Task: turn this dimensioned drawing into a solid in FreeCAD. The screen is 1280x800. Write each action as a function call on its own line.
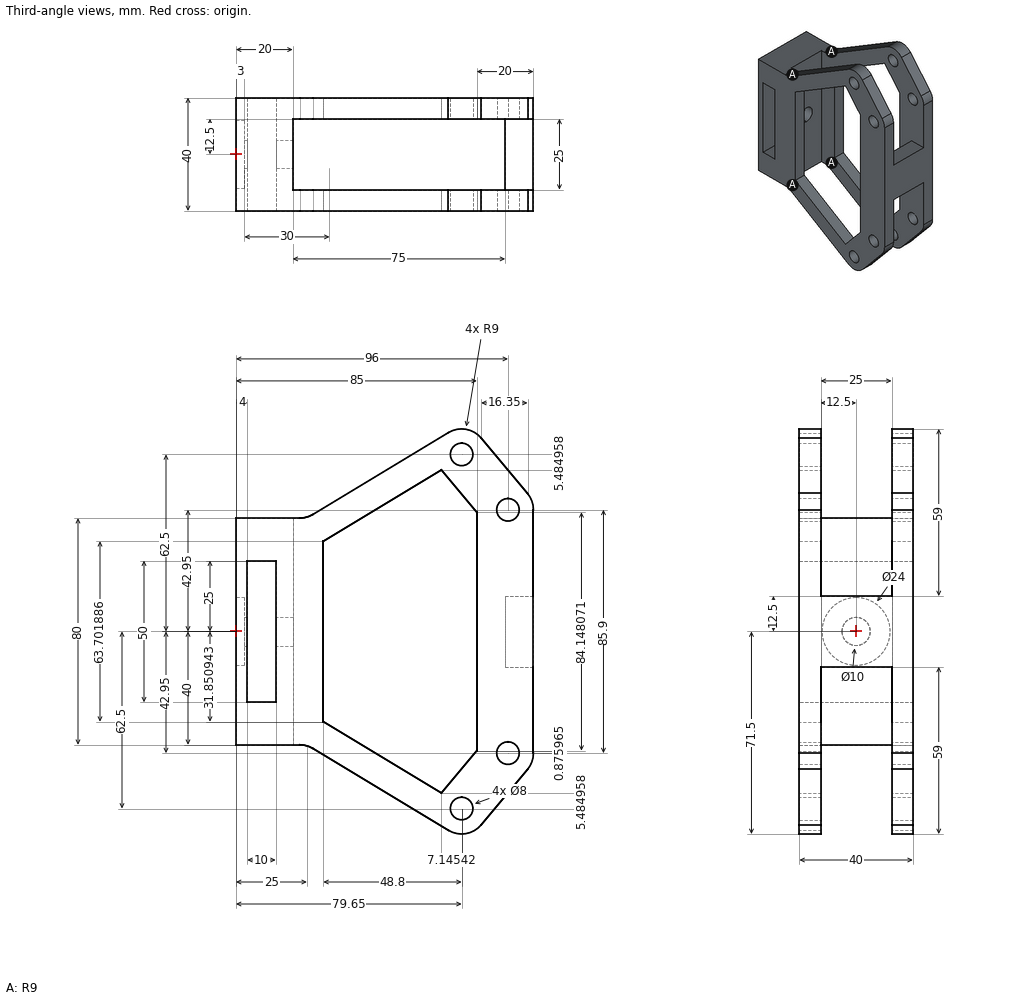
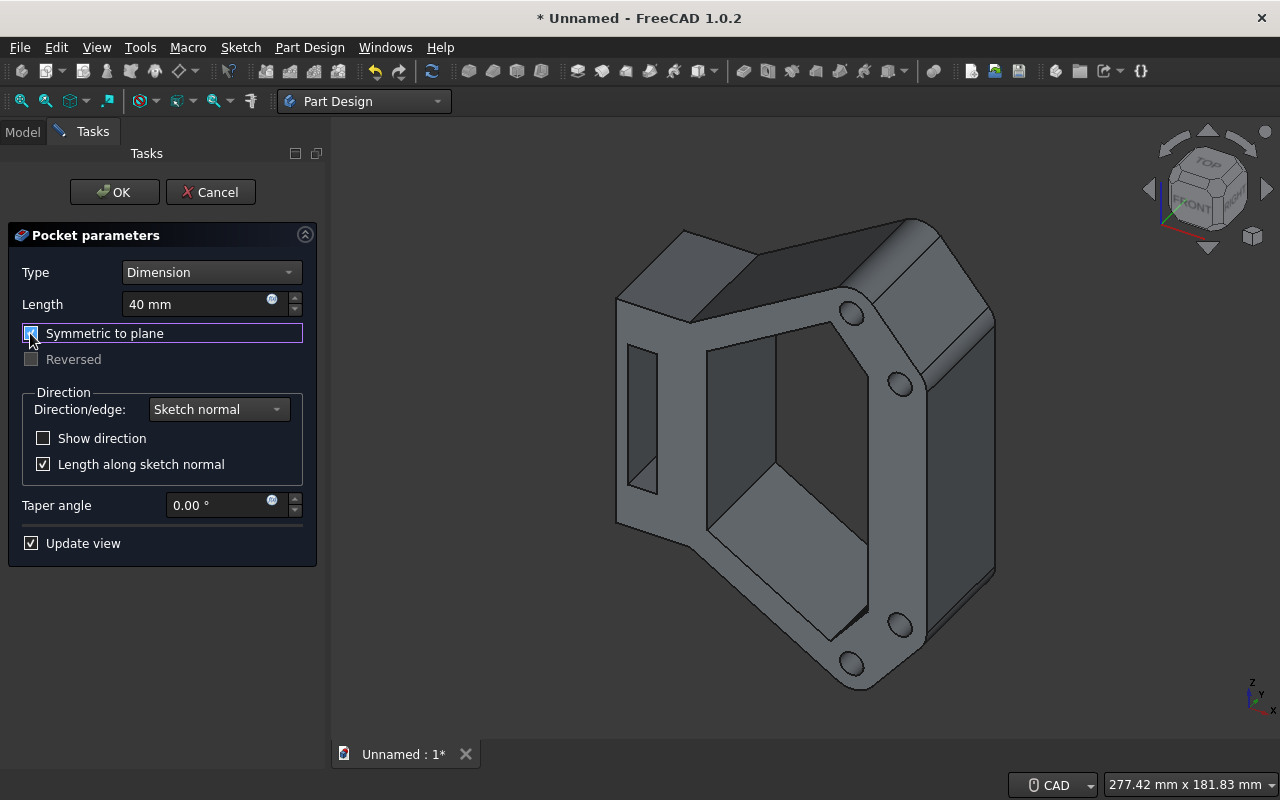
click(115, 192)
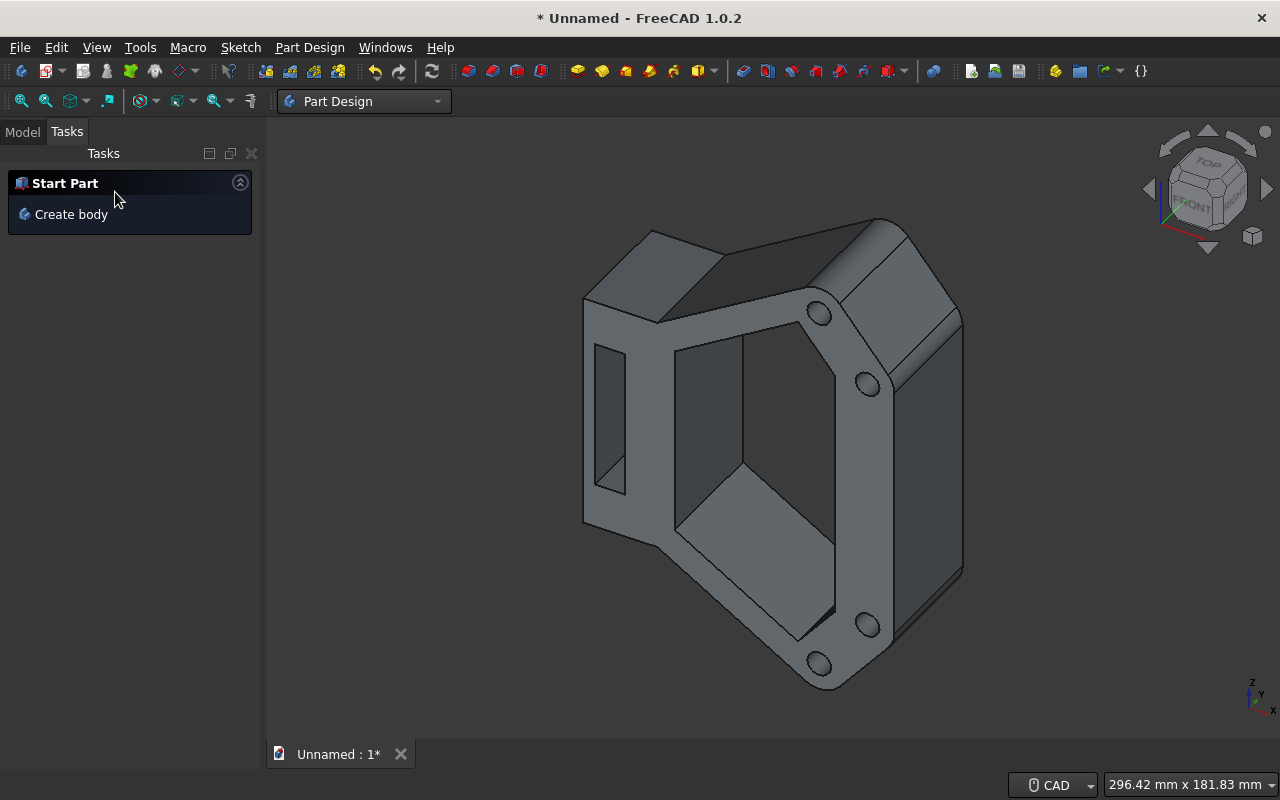
click(46, 72)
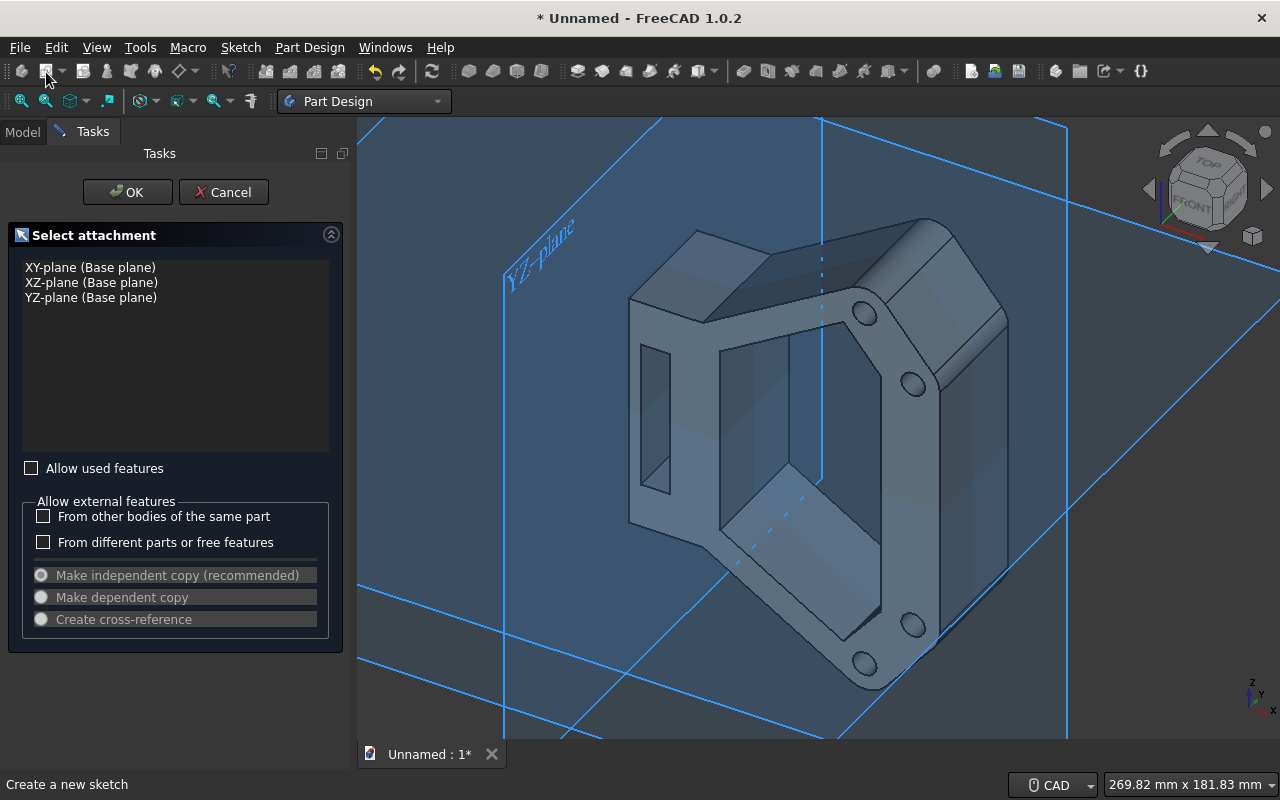
click(82, 268)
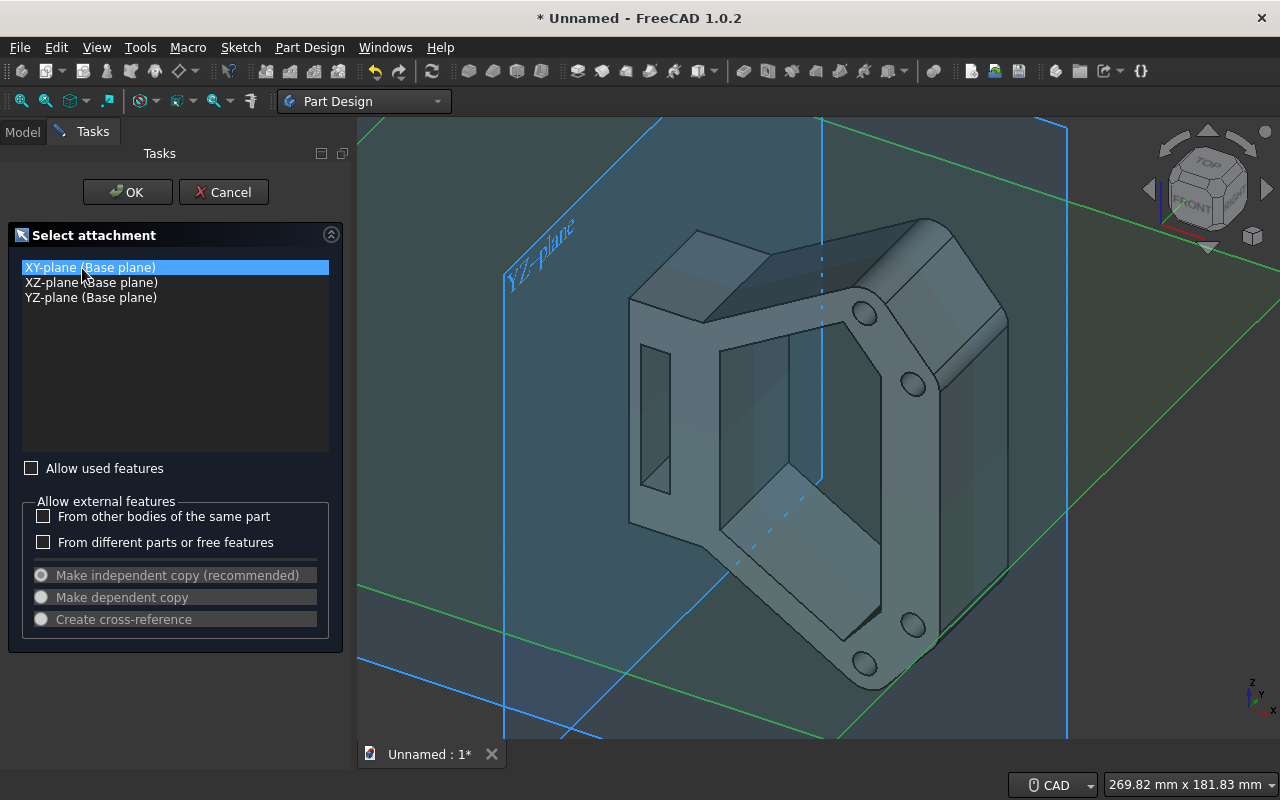
click(128, 192)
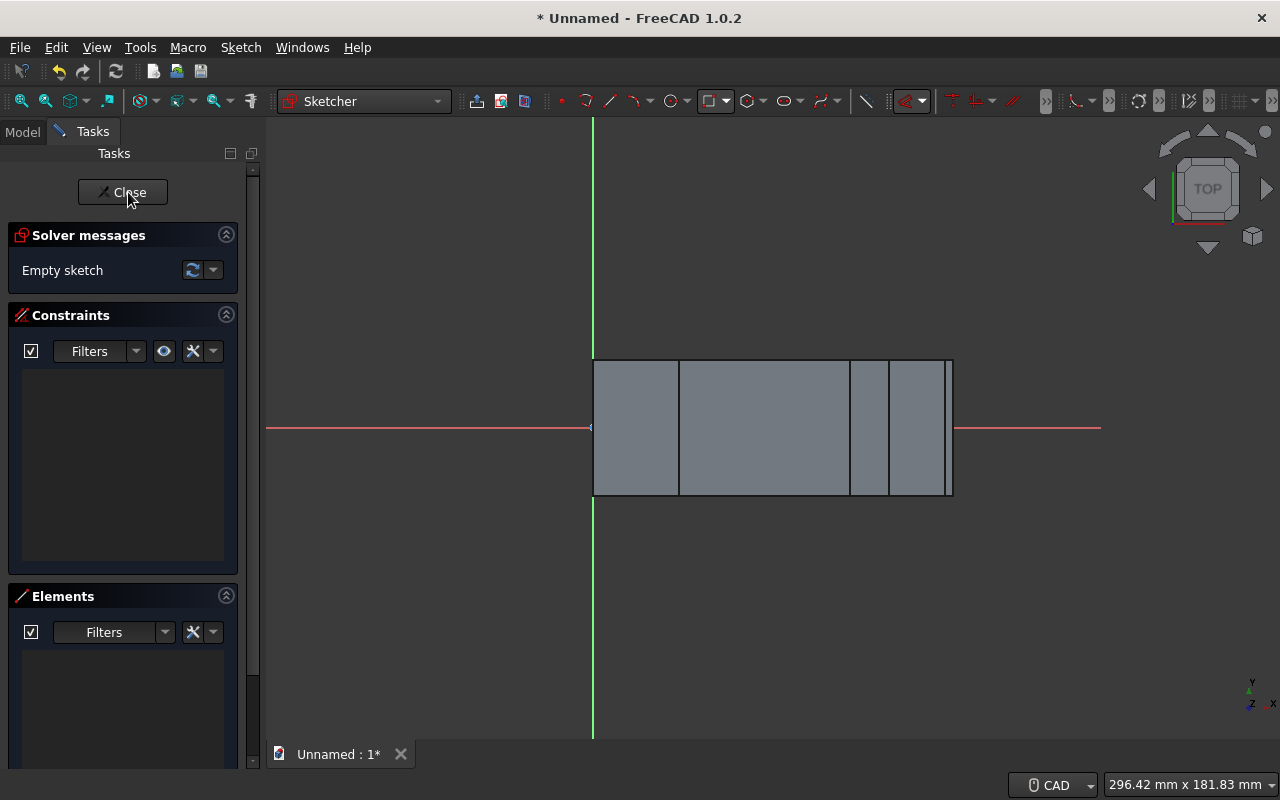
key(q)
key(s)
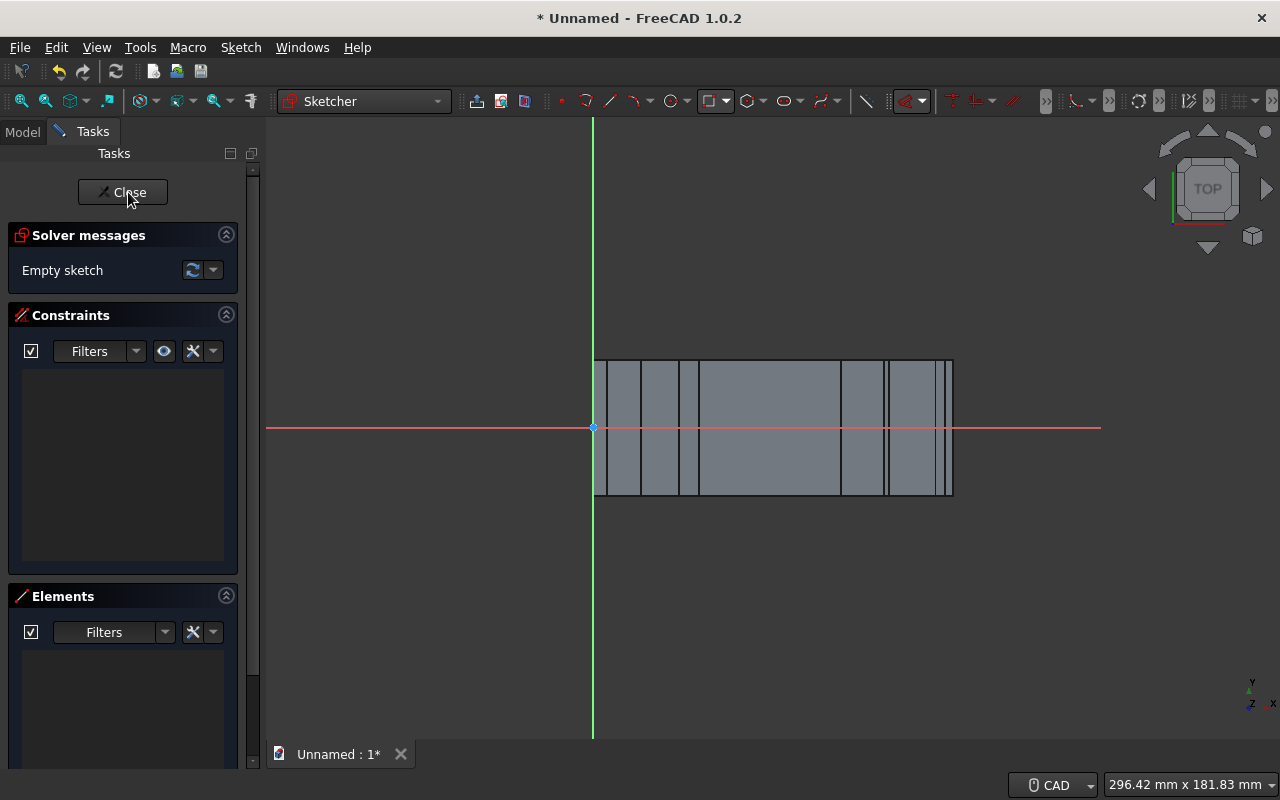
scroll(818, 428, up, 3)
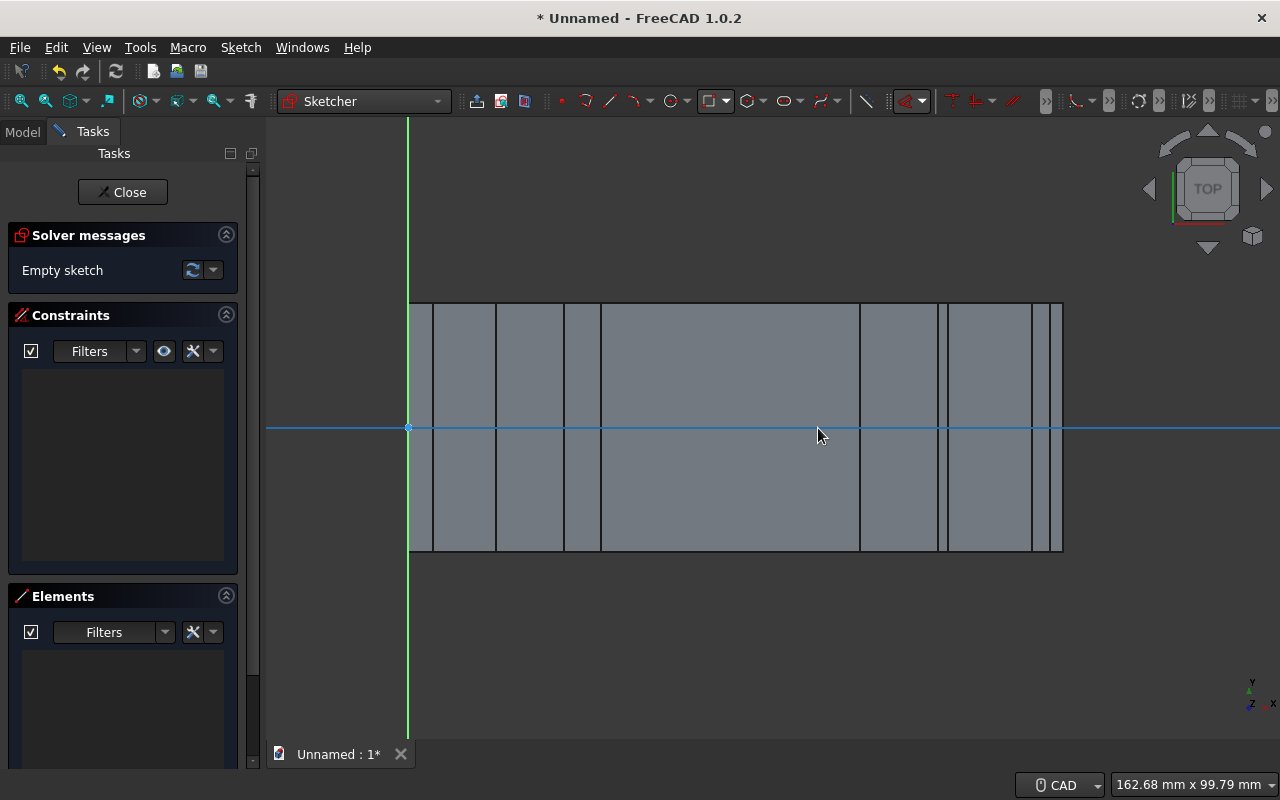
key(g)
key(r)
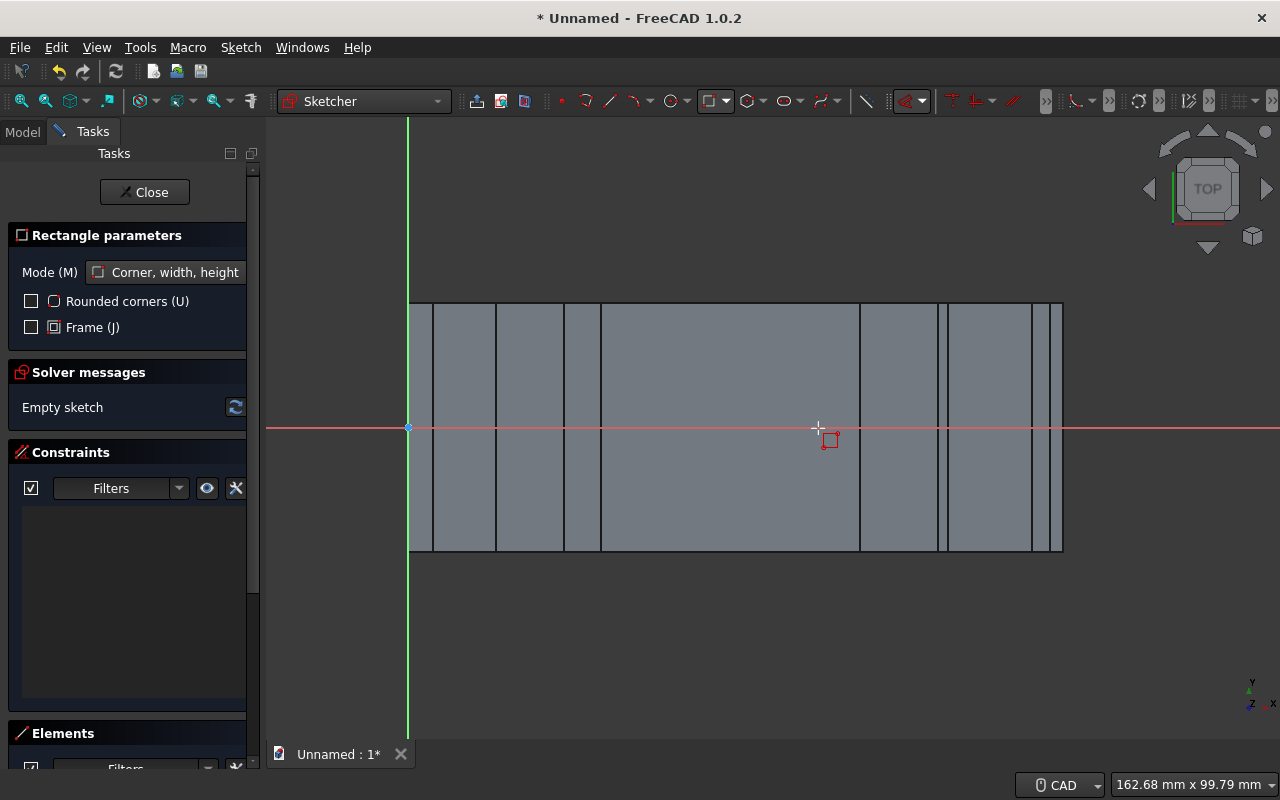
click(533, 350)
move(1000, 506)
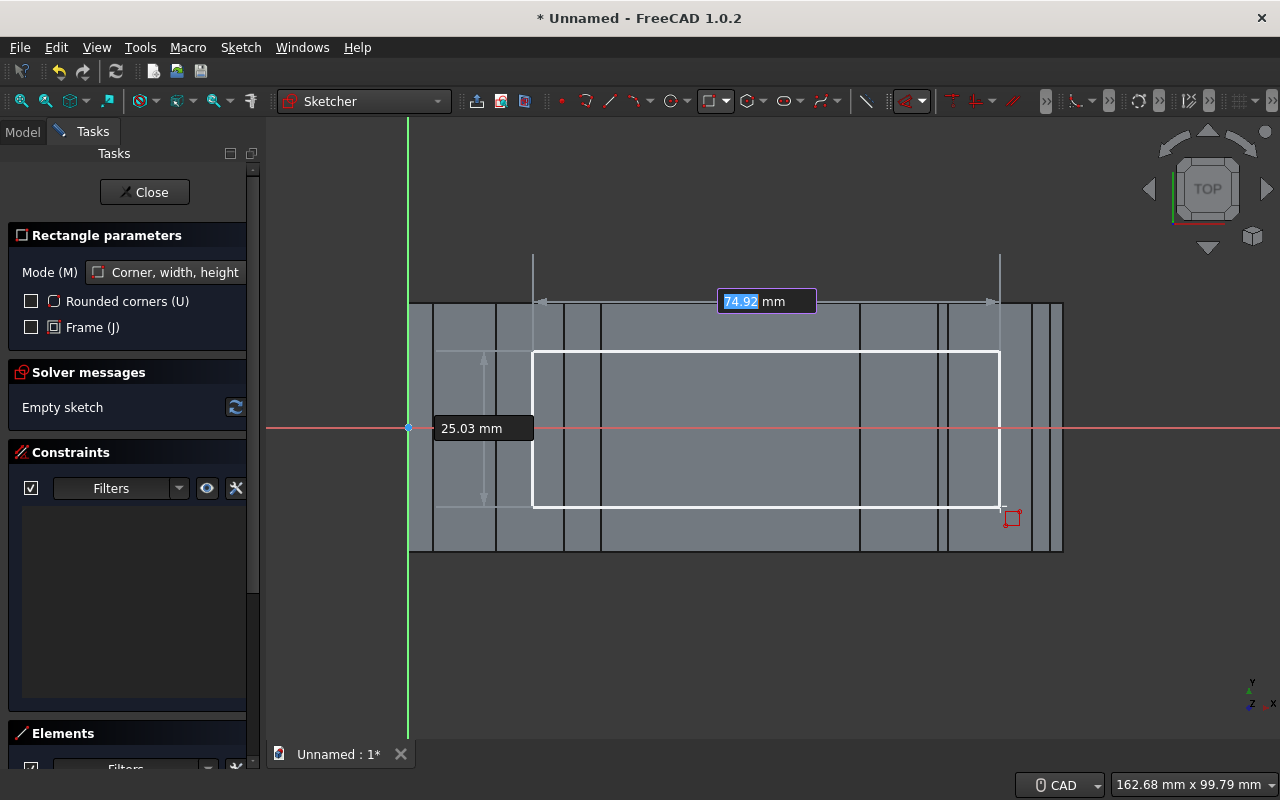
text(75)
key(Tab)
text(25)
key(Return)
key(Escape)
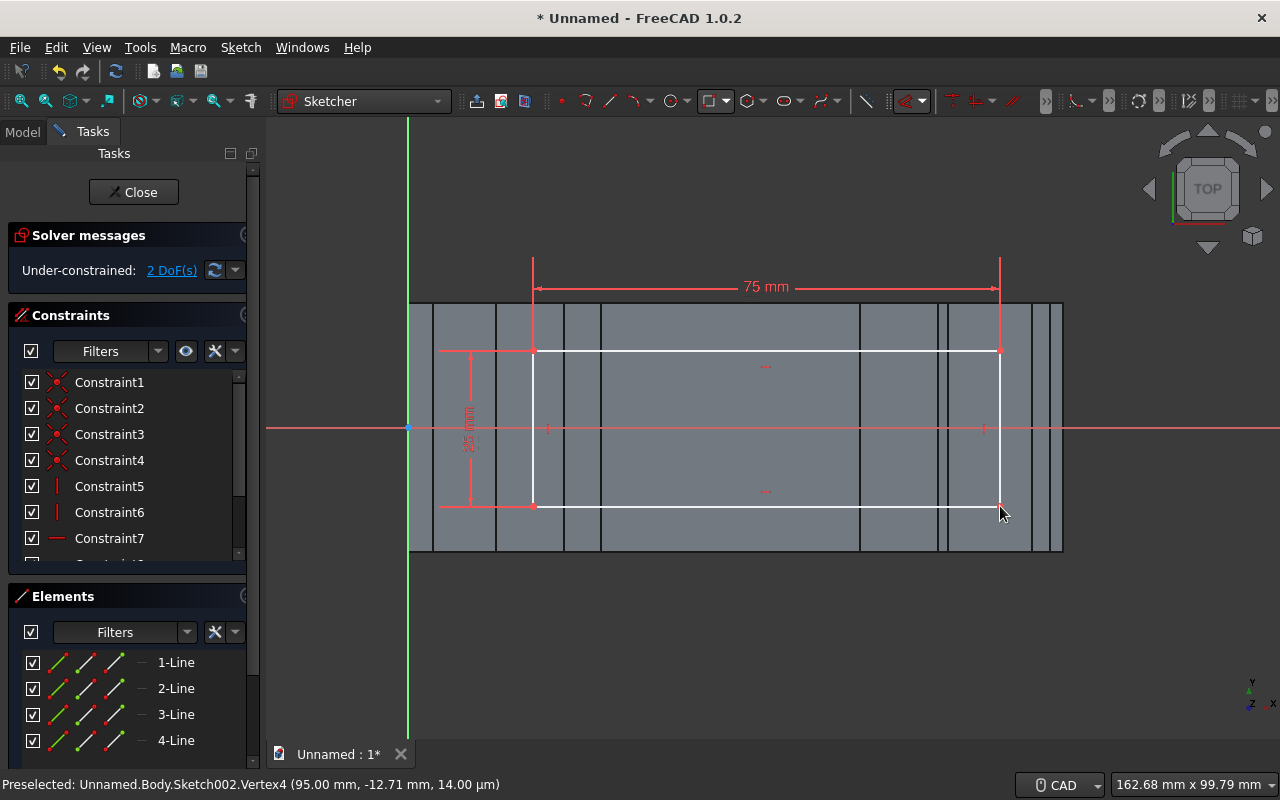
click(533, 351)